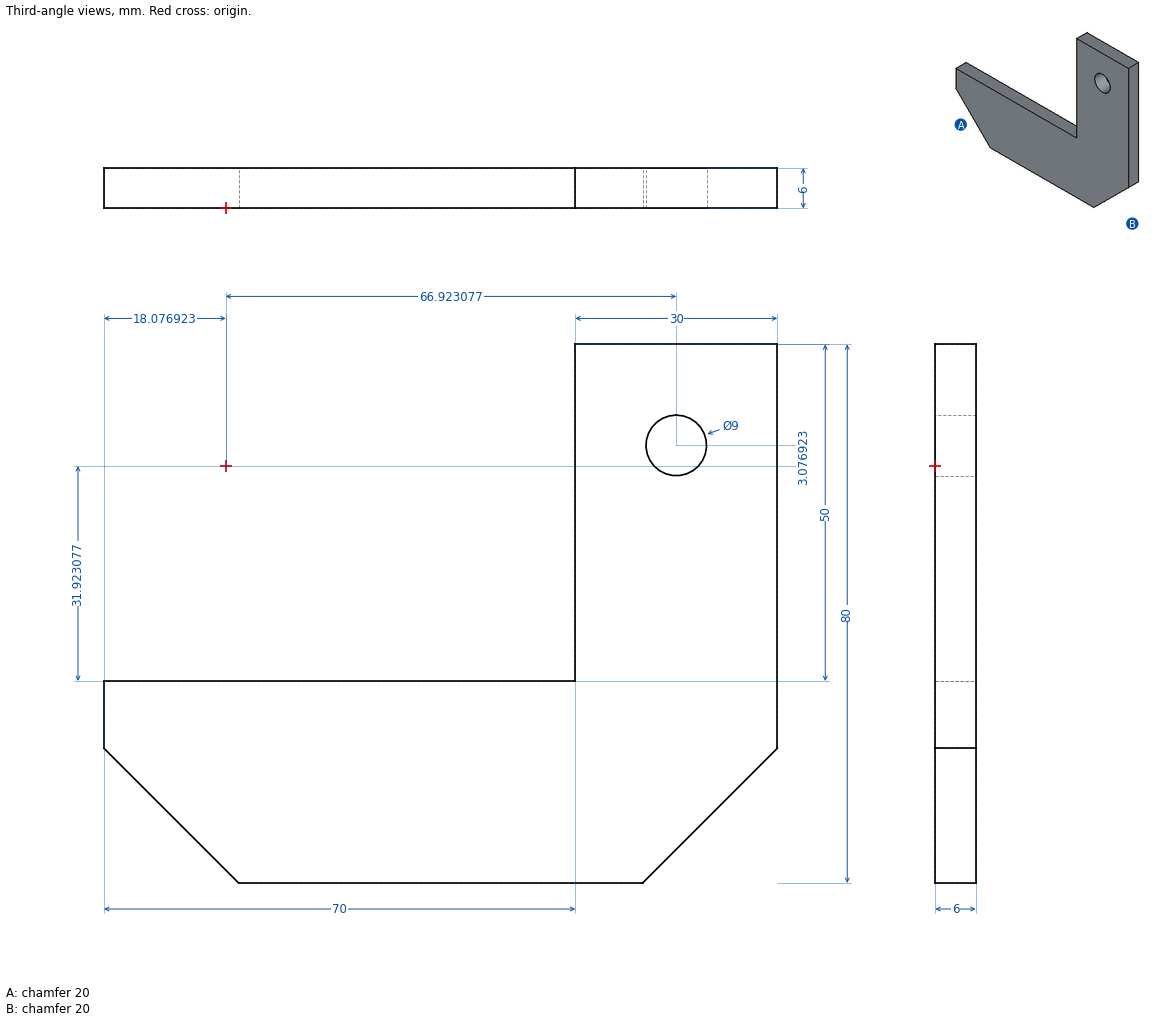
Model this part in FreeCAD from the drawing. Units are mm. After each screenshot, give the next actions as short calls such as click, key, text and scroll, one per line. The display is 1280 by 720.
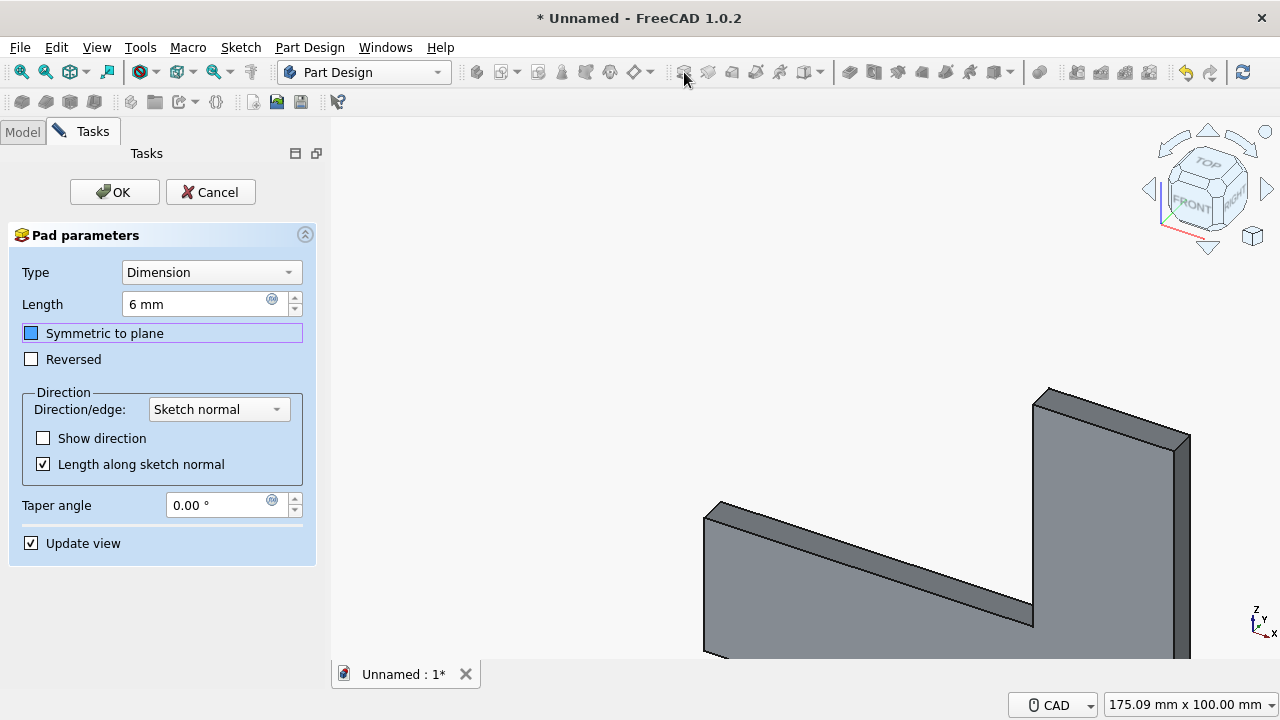
click(30, 359)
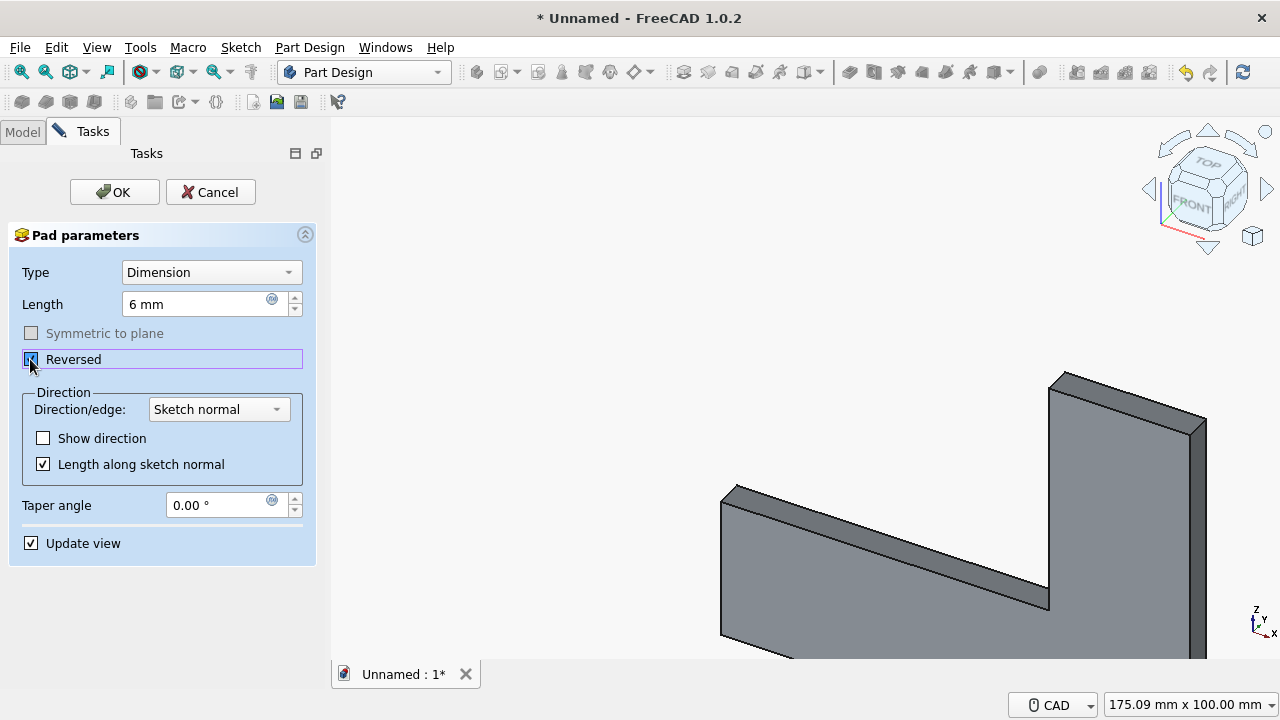
click(115, 192)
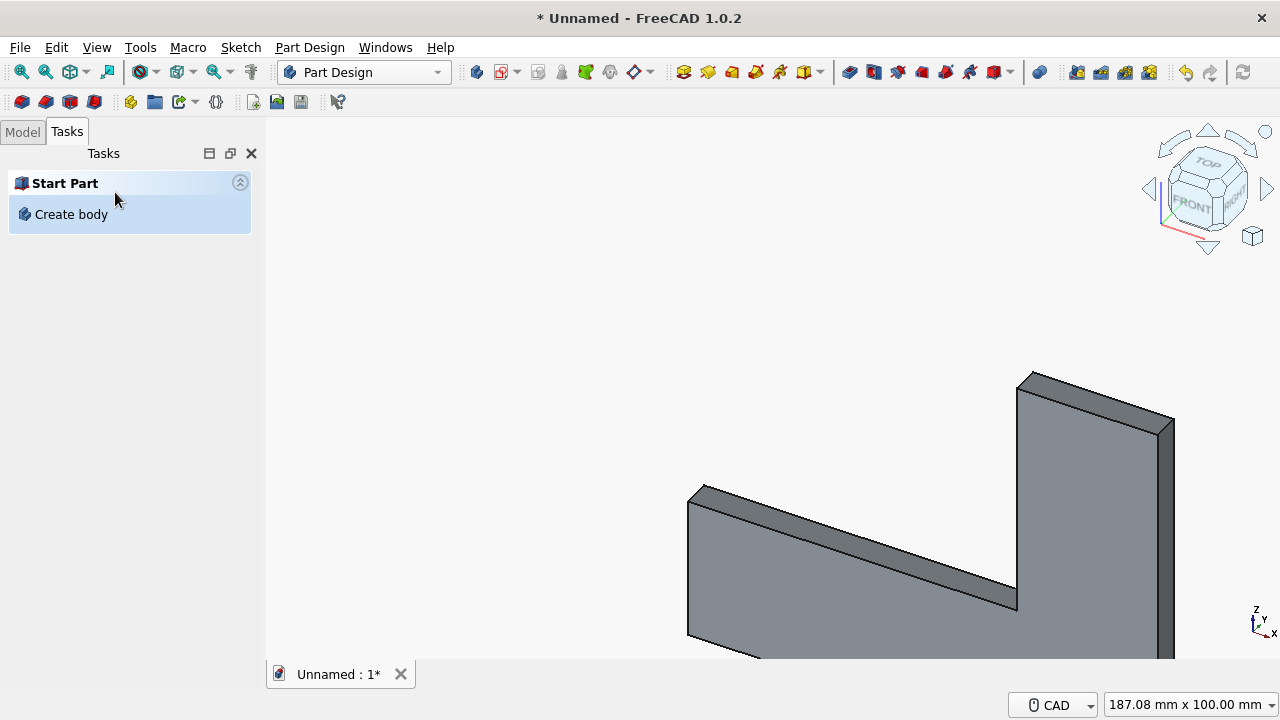
click(22, 72)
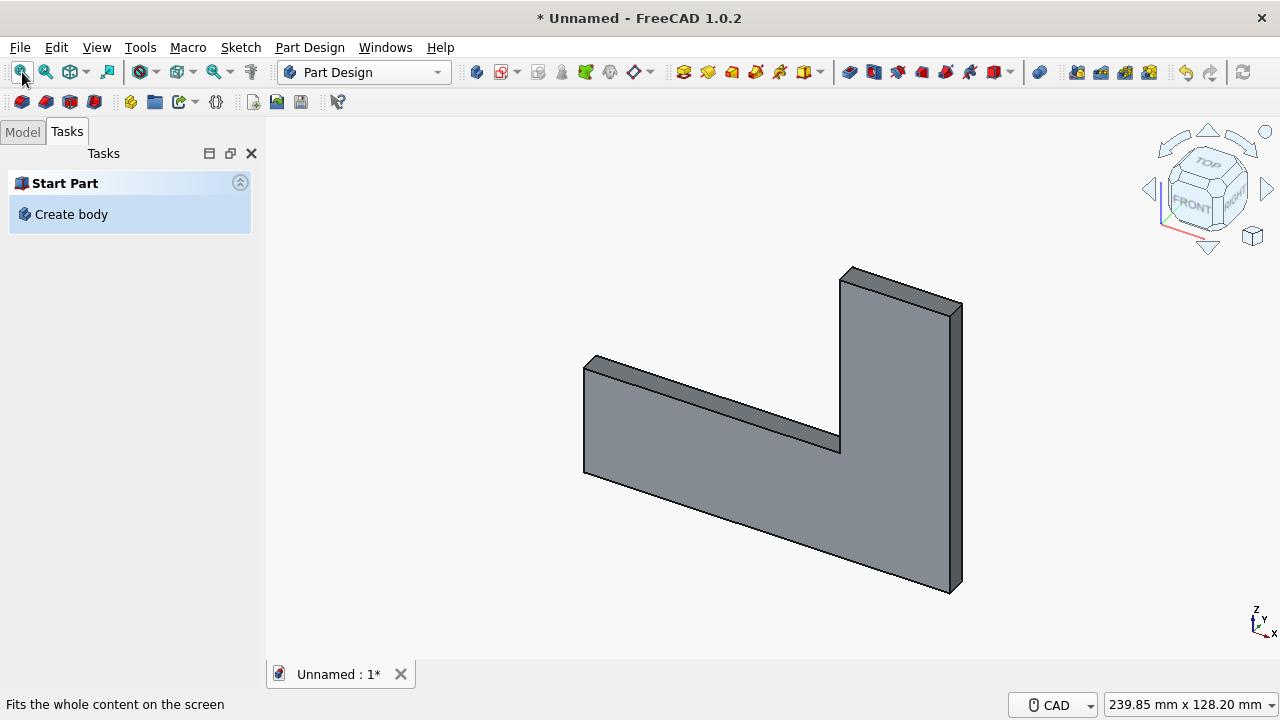
key(4)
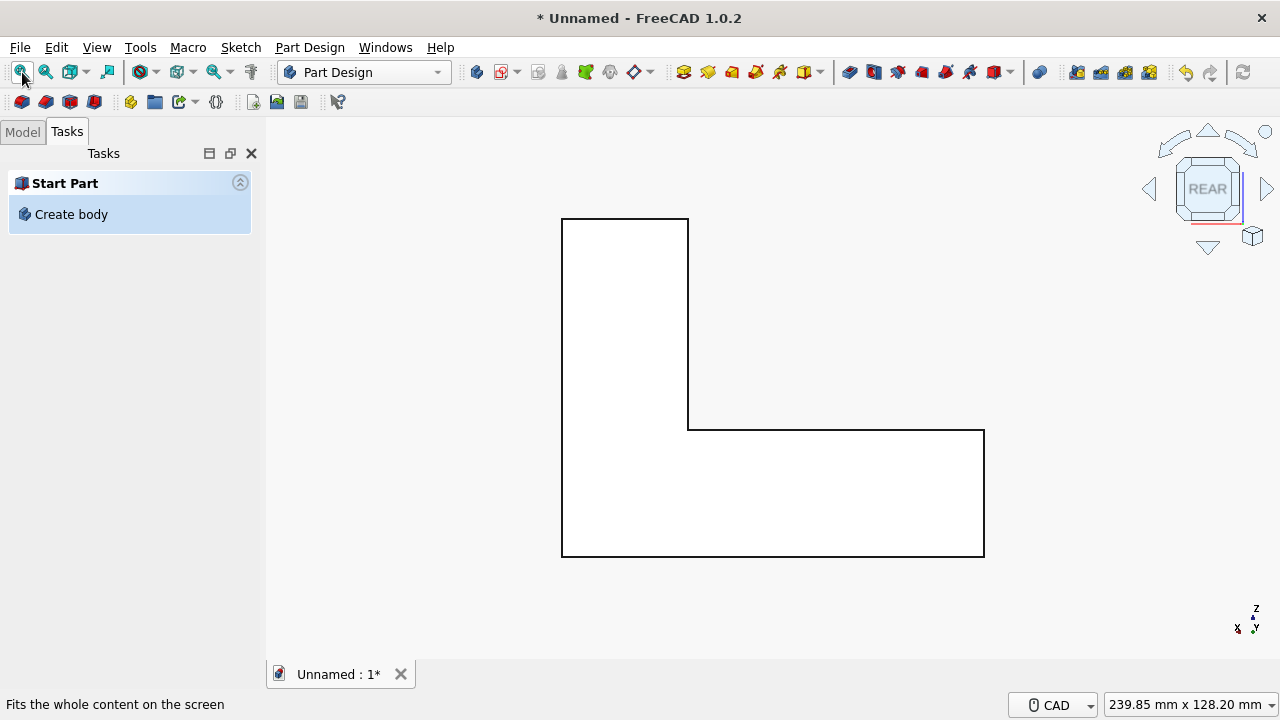
click(652, 484)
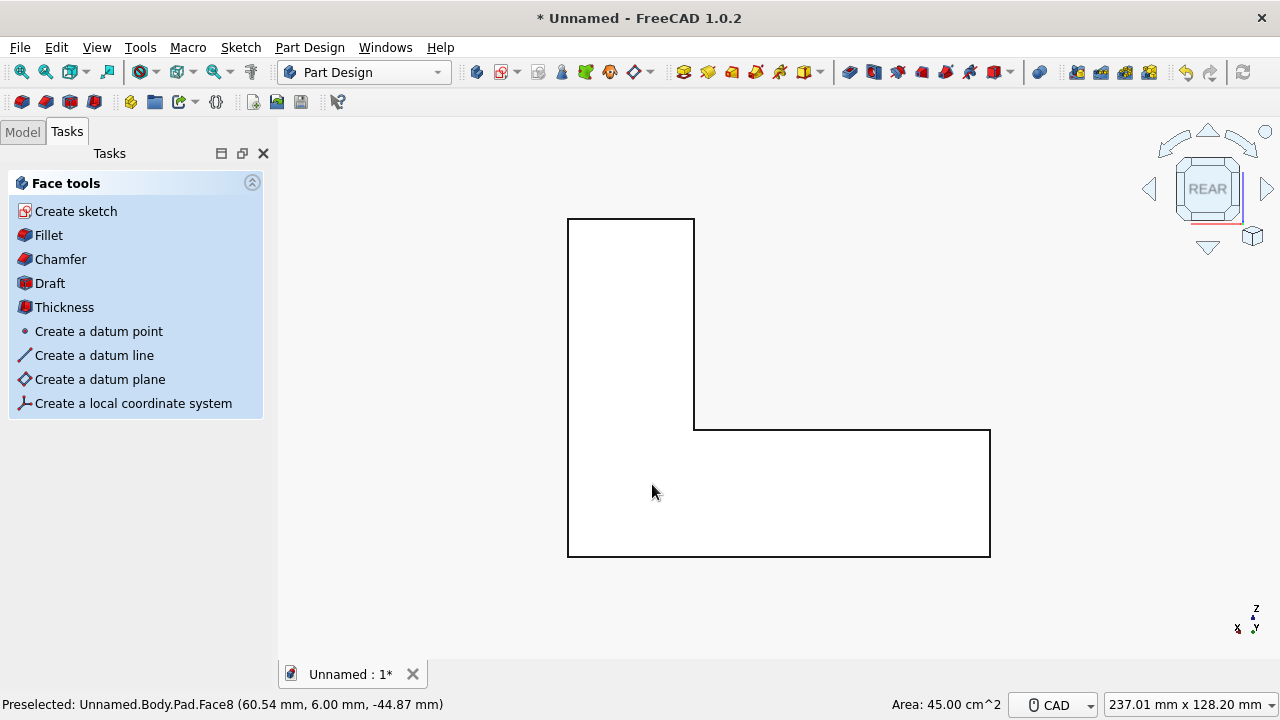
click(502, 72)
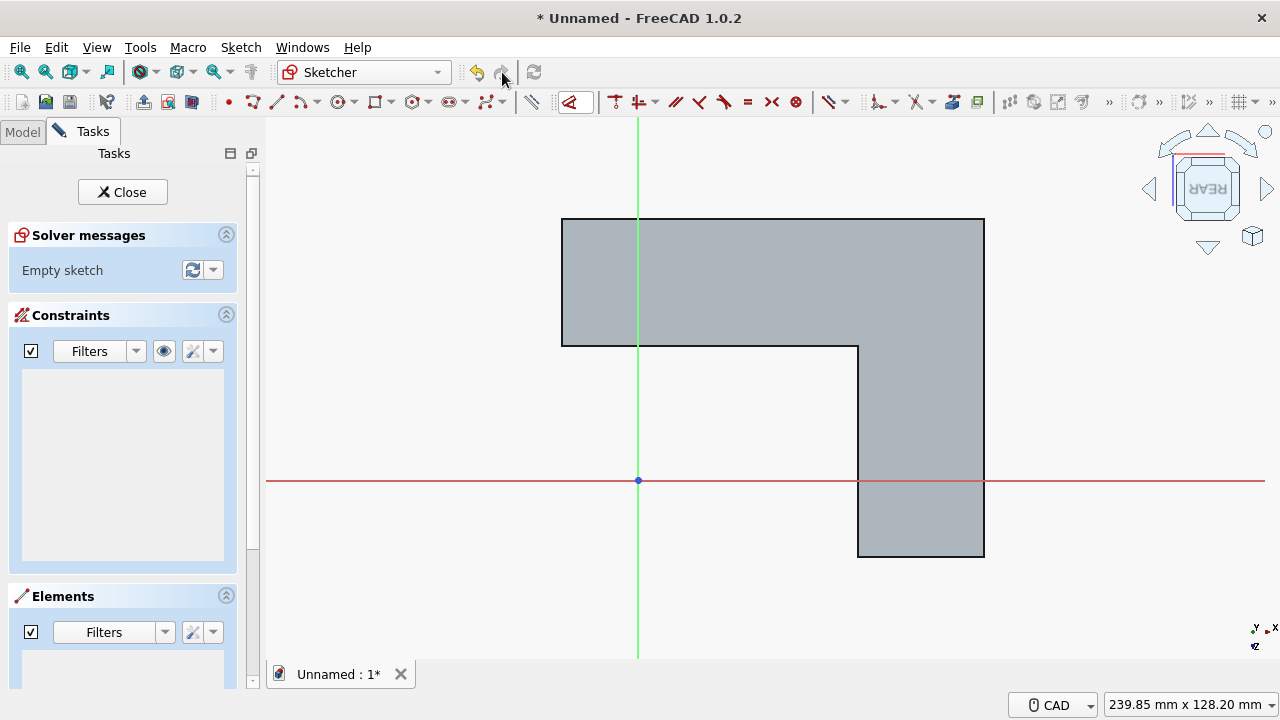
scroll(948, 507, up, 11)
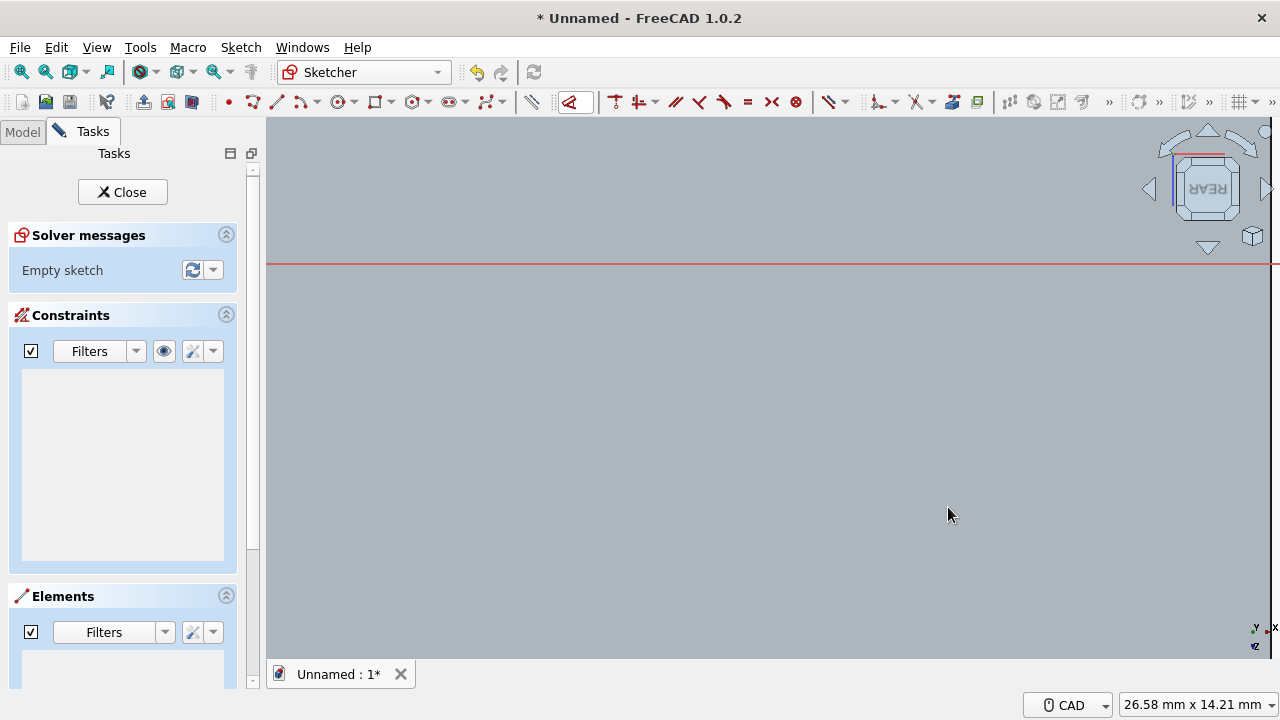
key(g)
key(c)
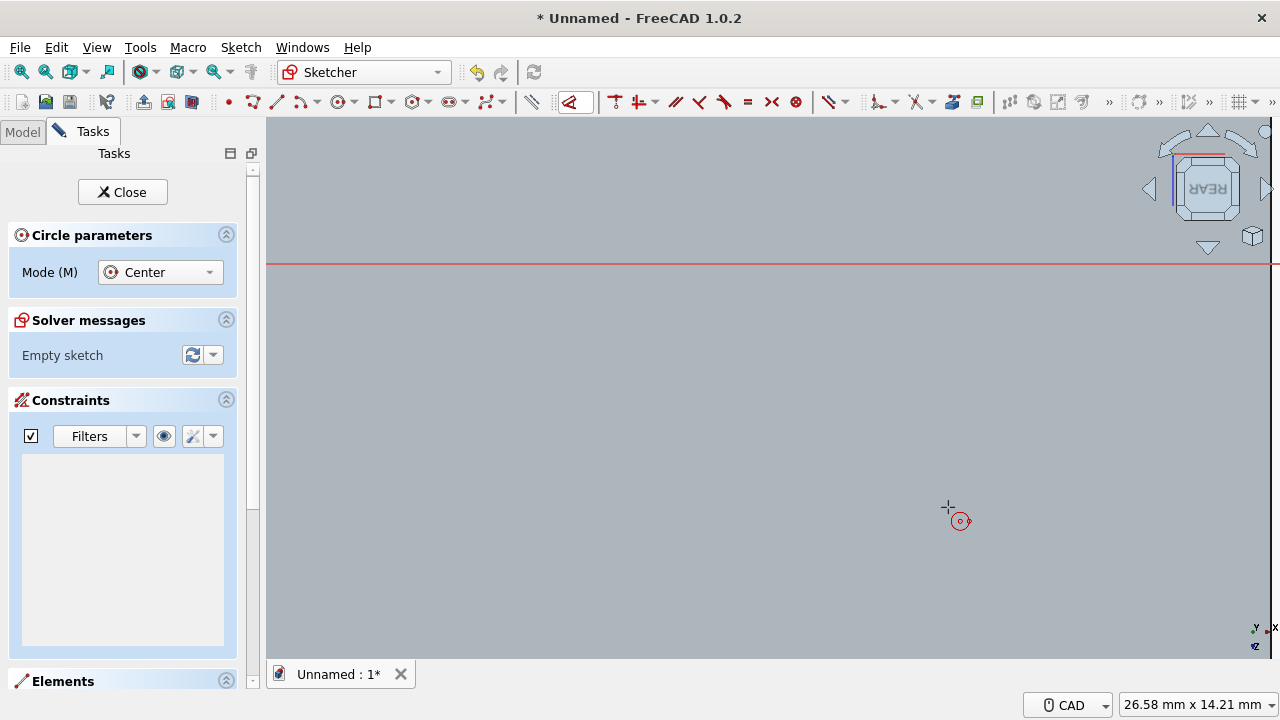
click(699, 381)
move(820, 503)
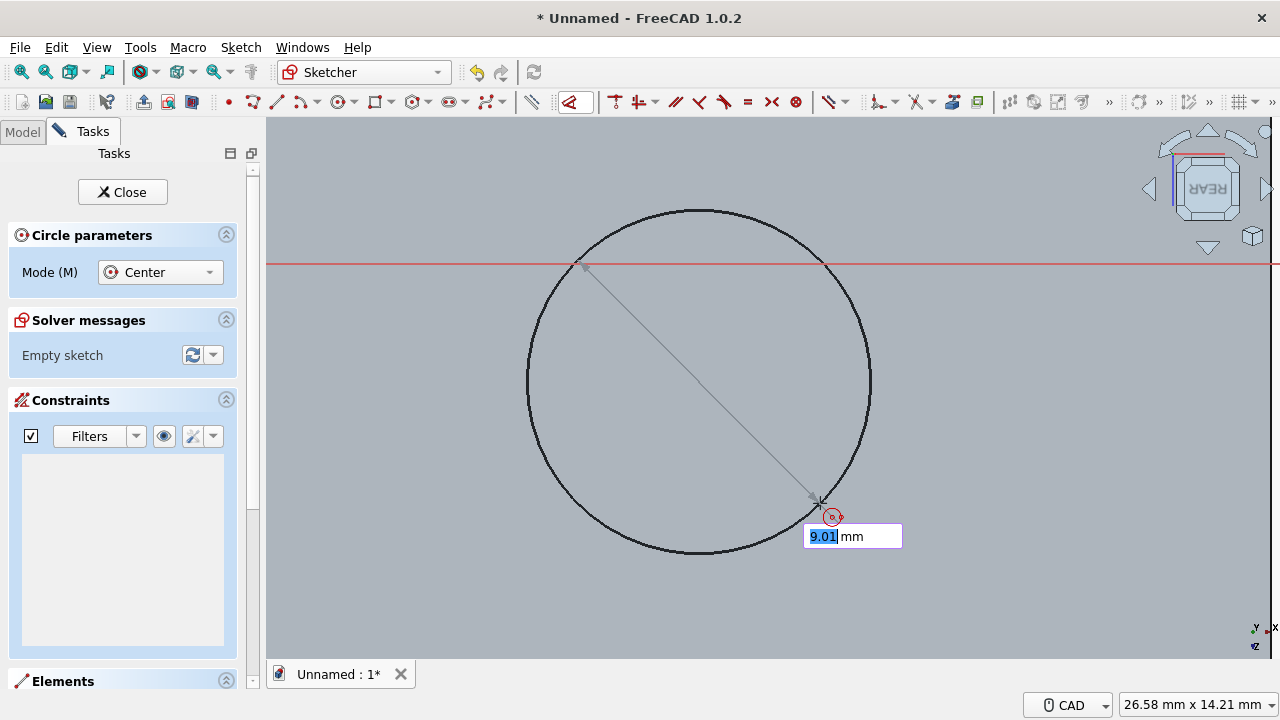
text(9)
key(Return)
key(Escape)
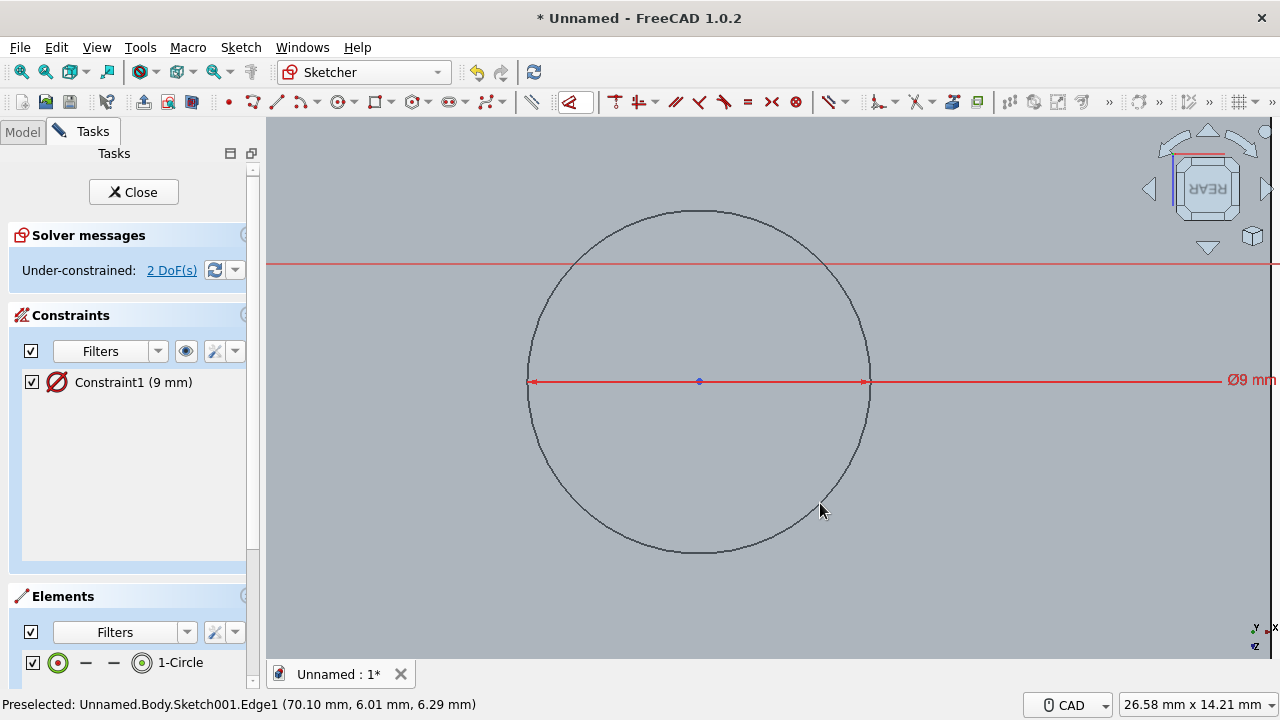
click(699, 382)